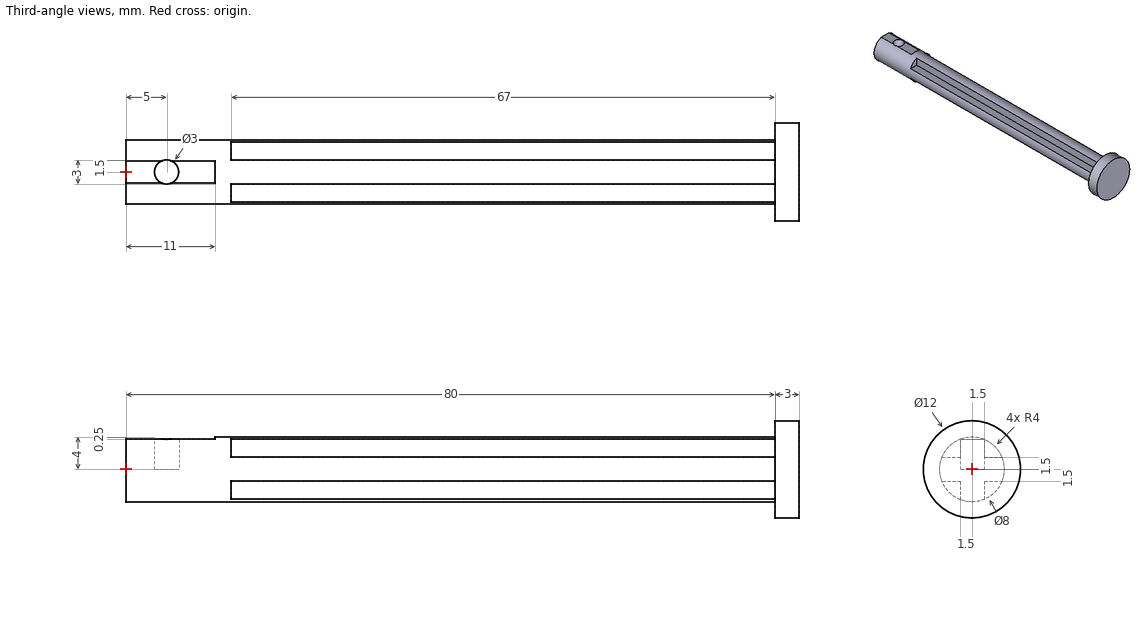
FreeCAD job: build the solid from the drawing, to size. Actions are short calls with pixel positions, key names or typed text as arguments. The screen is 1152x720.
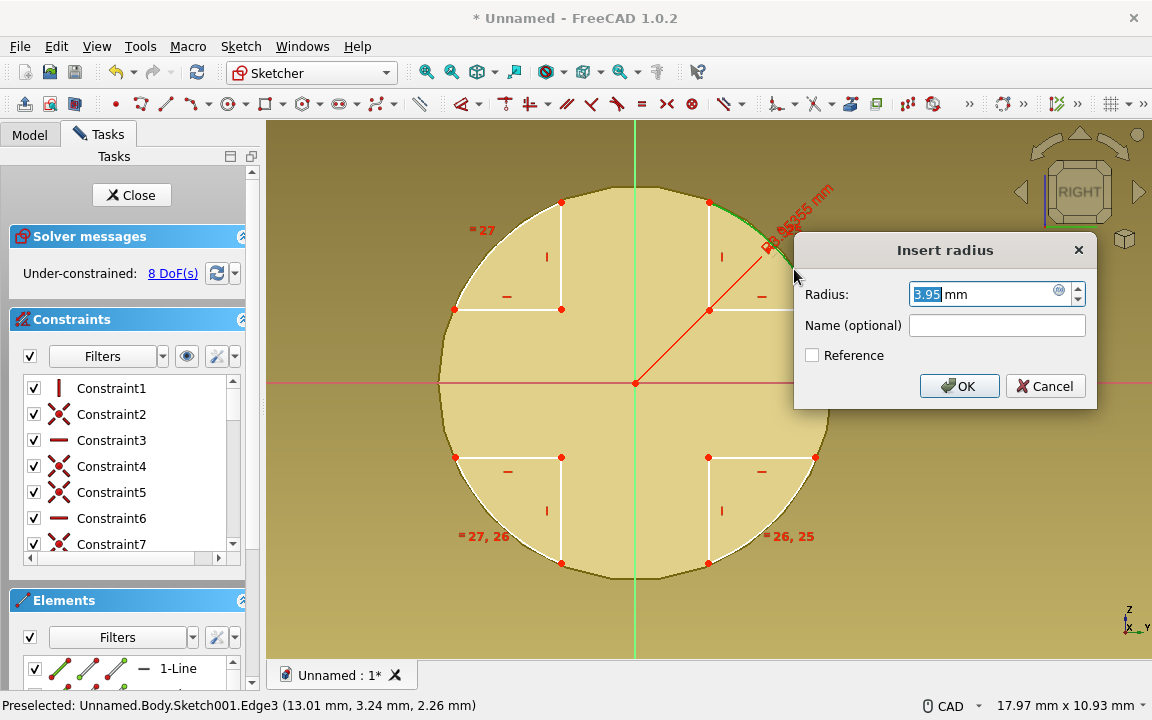
text(4)
key(Return)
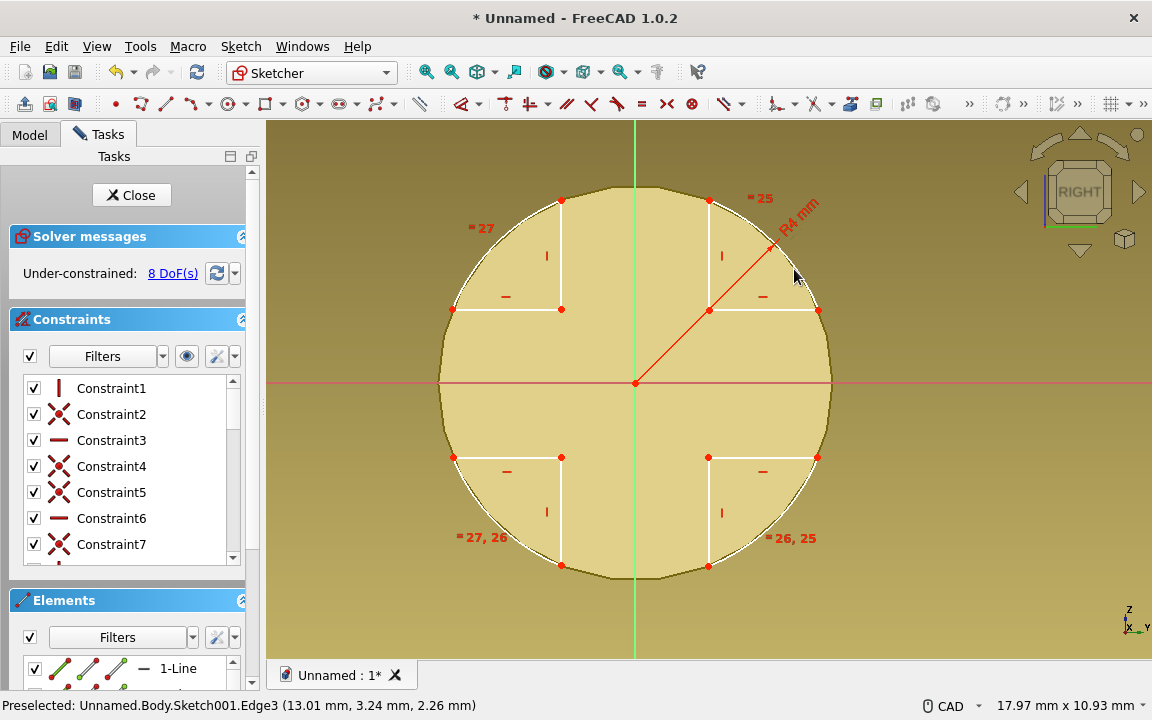
click(709, 200)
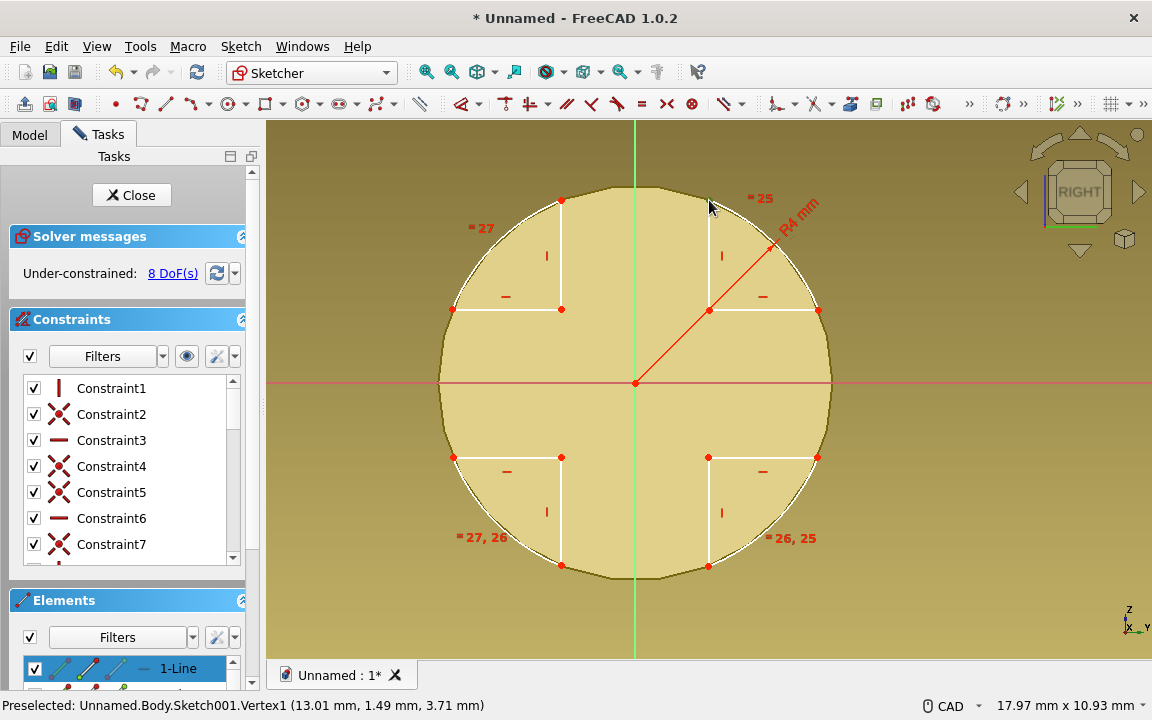
key(l)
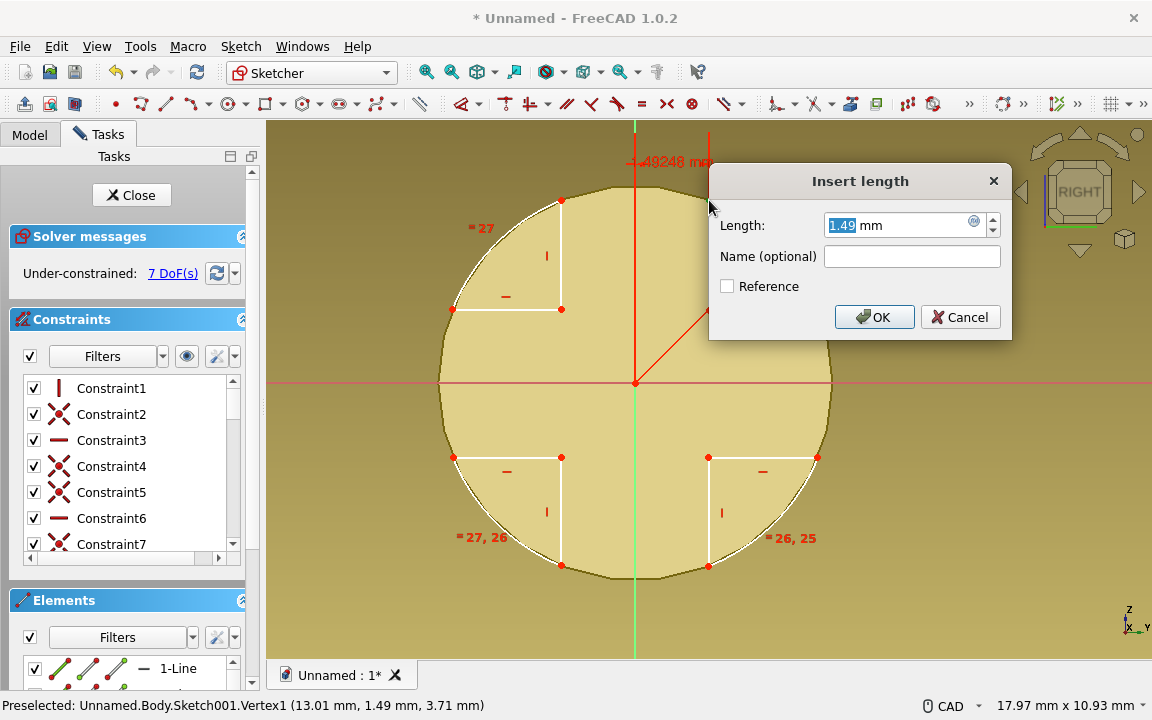
text(1.5)
key(Return)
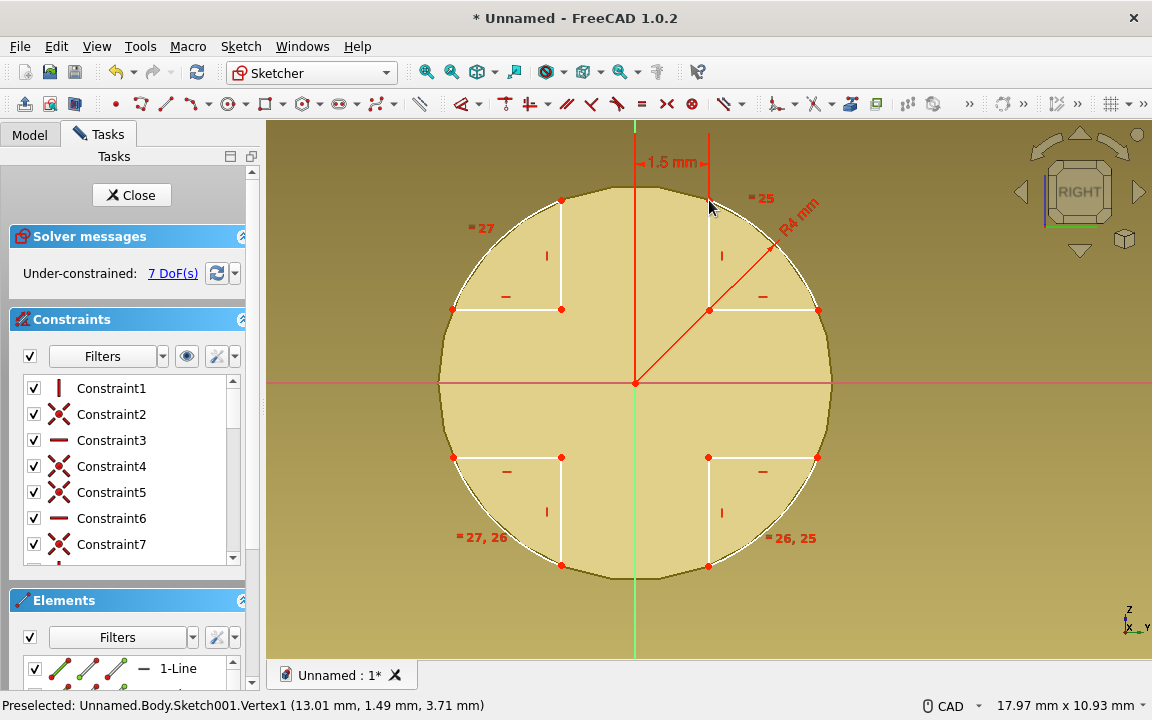
click(709, 310)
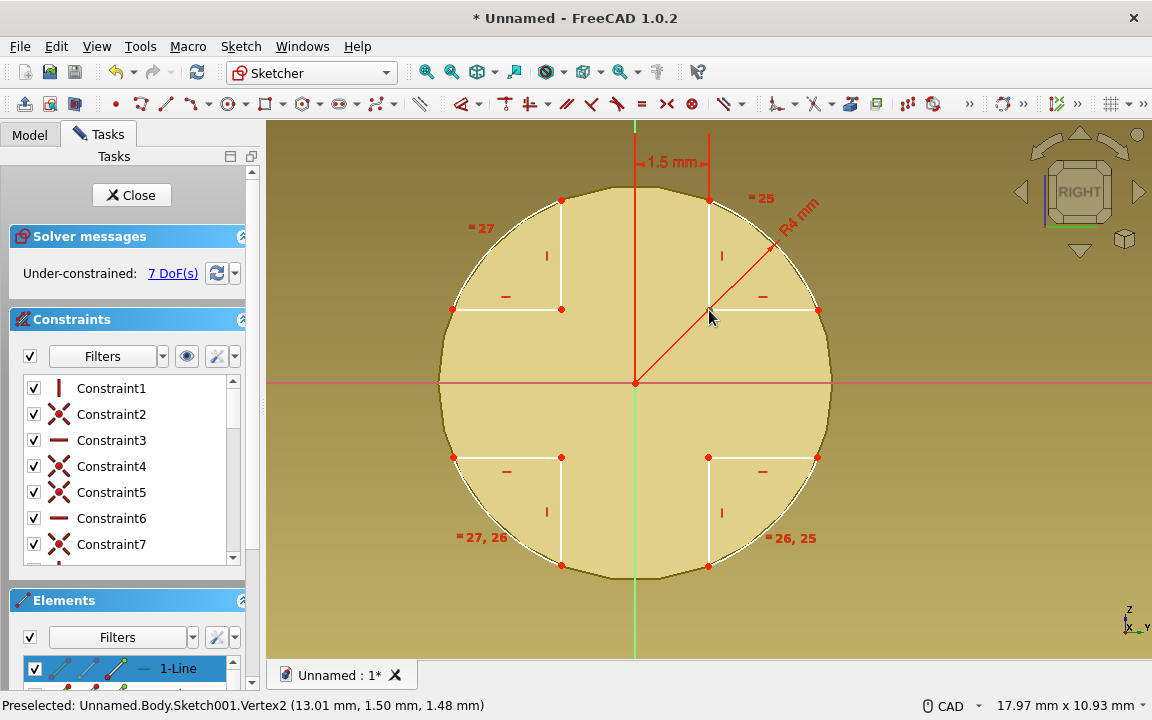
key(i)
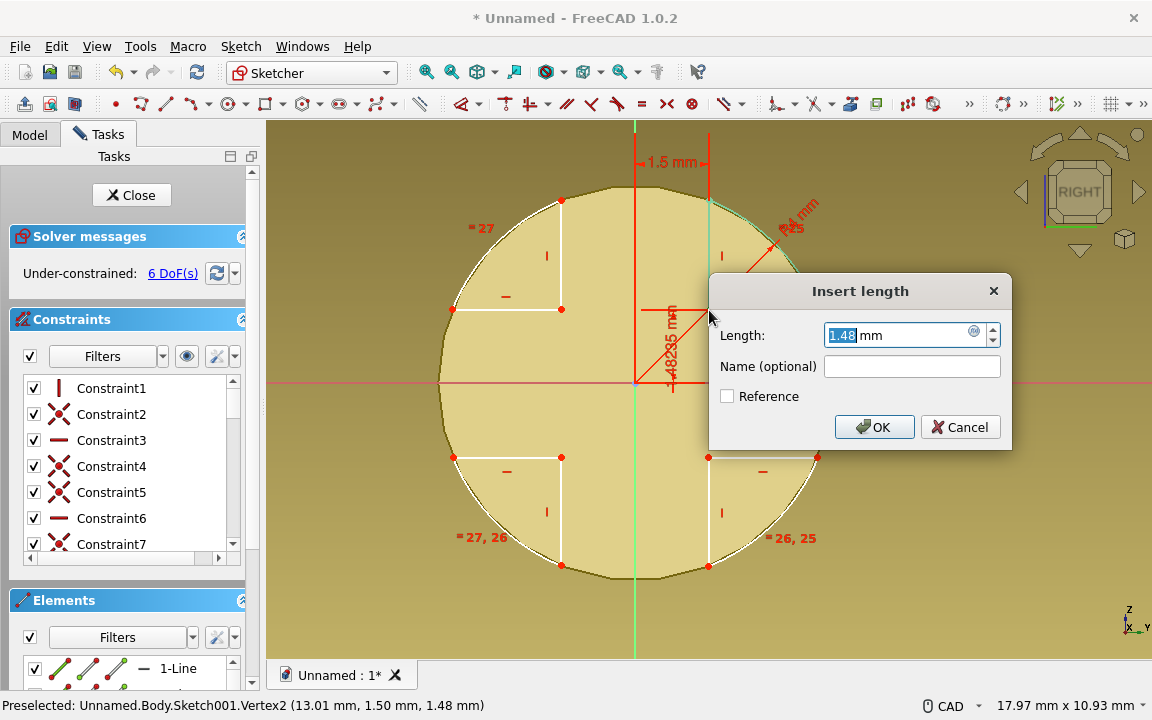
text(1.5)
key(Return)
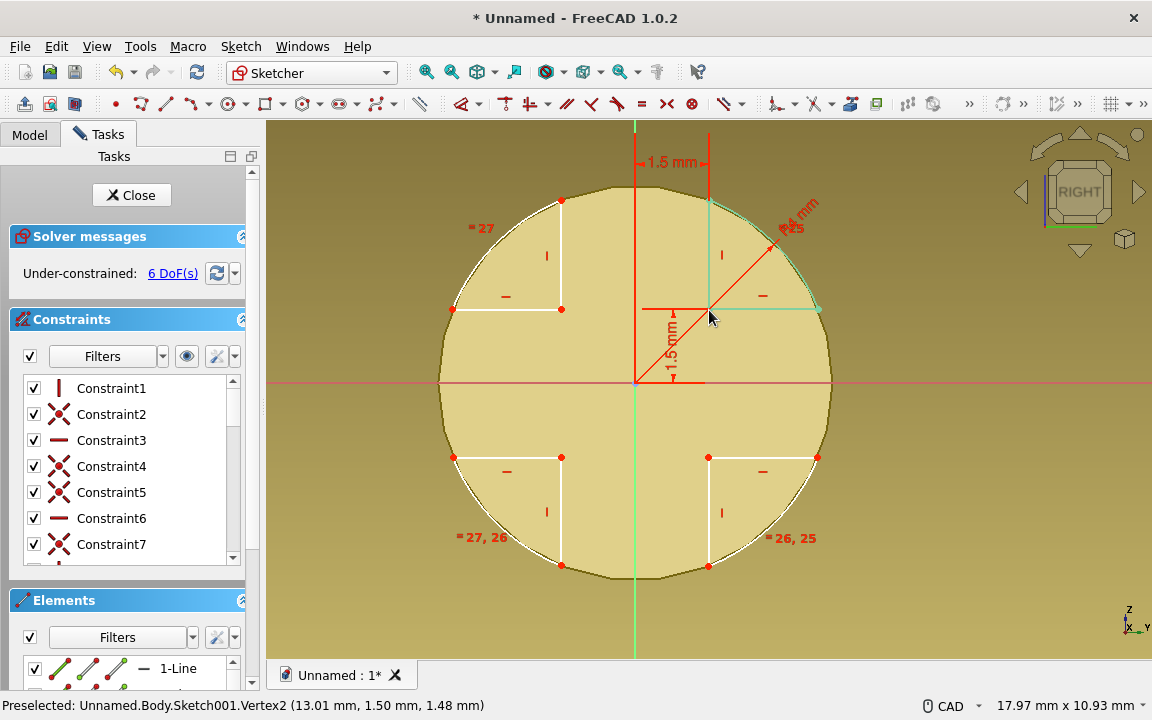
click(818, 458)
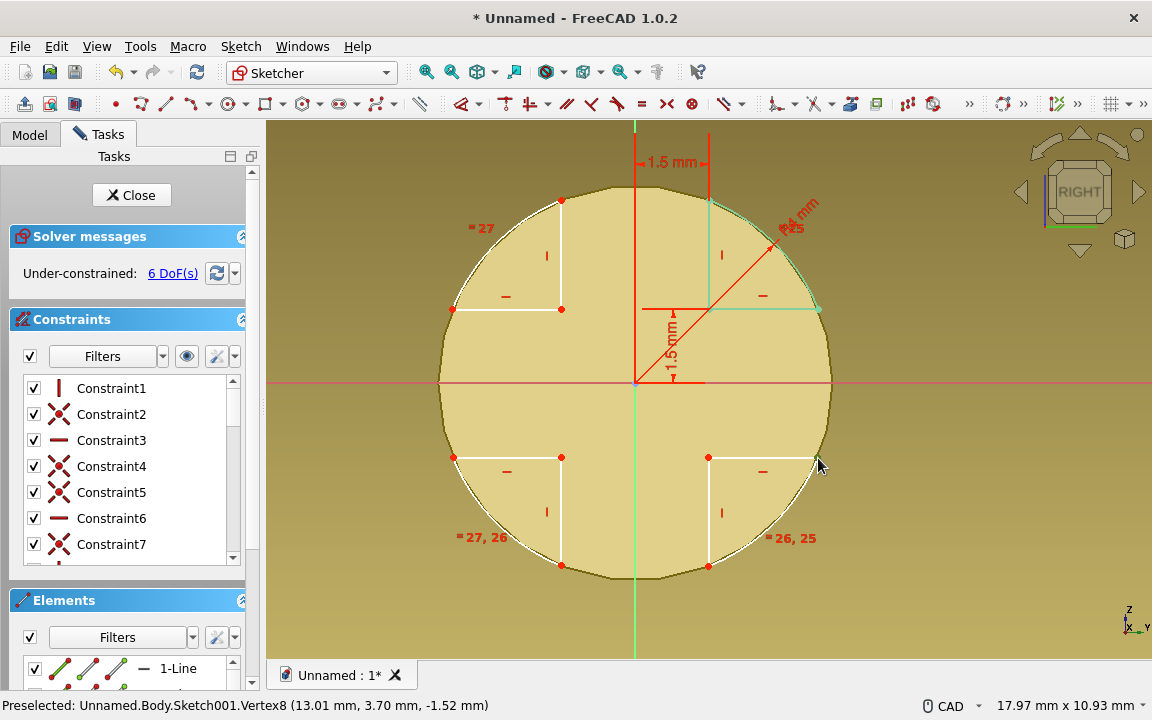
key(i)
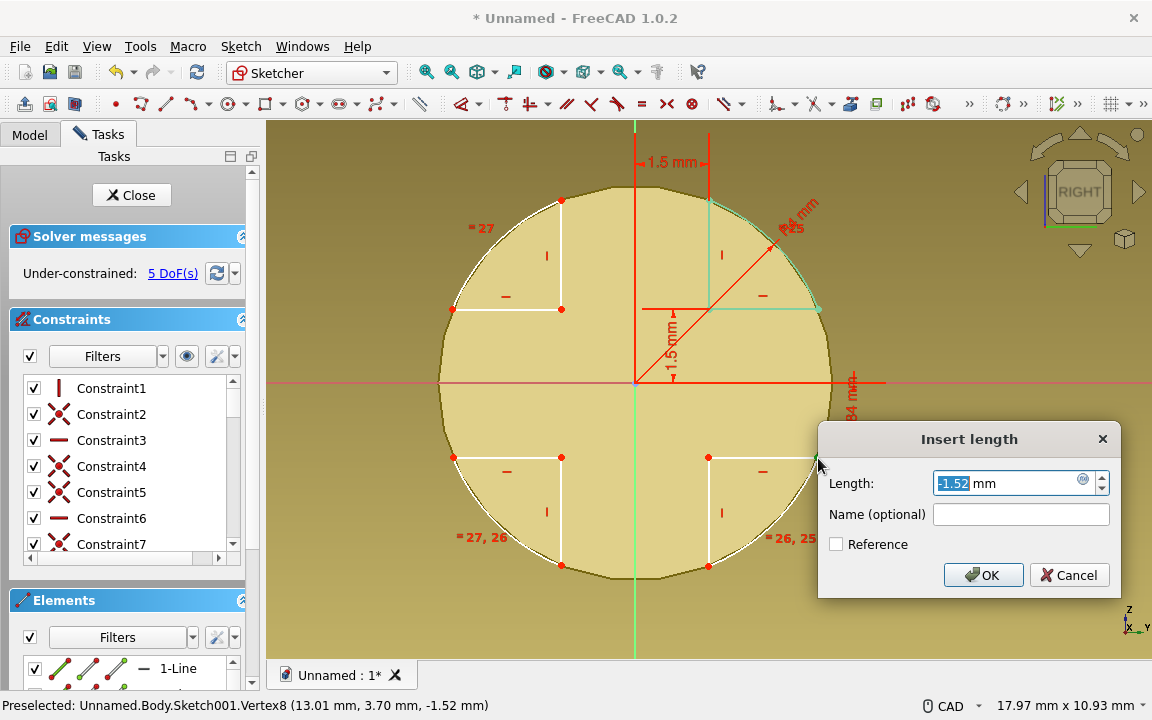
text(-1.5)
key(Return)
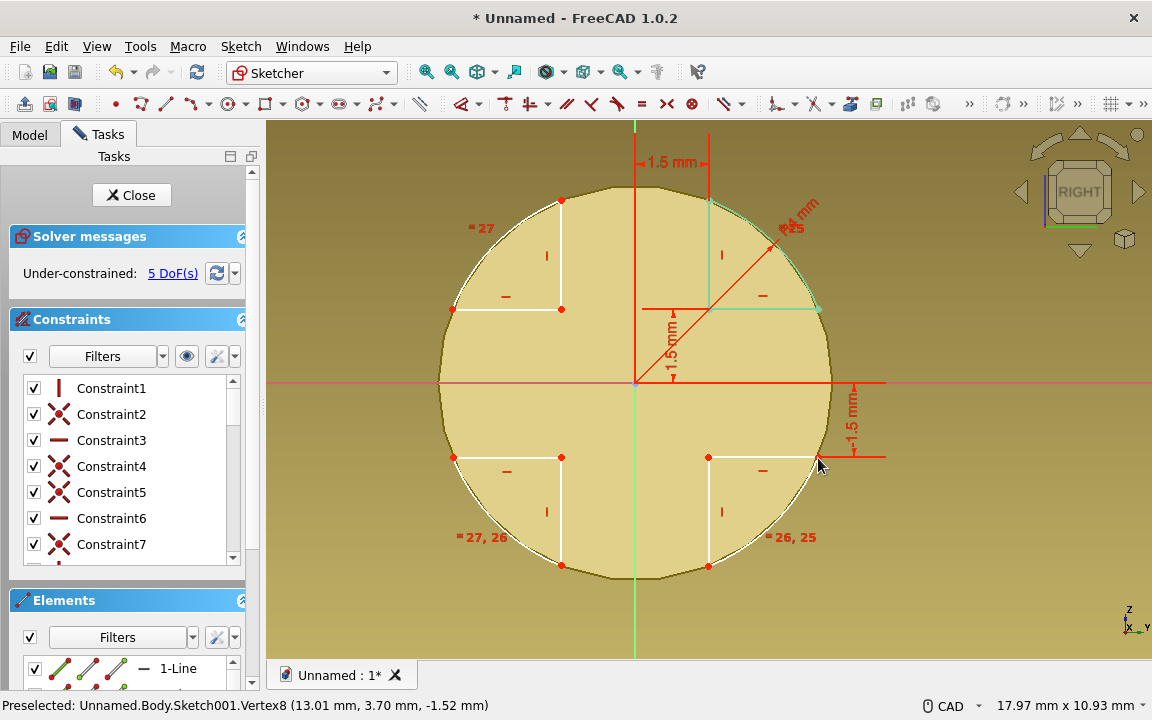
click(709, 457)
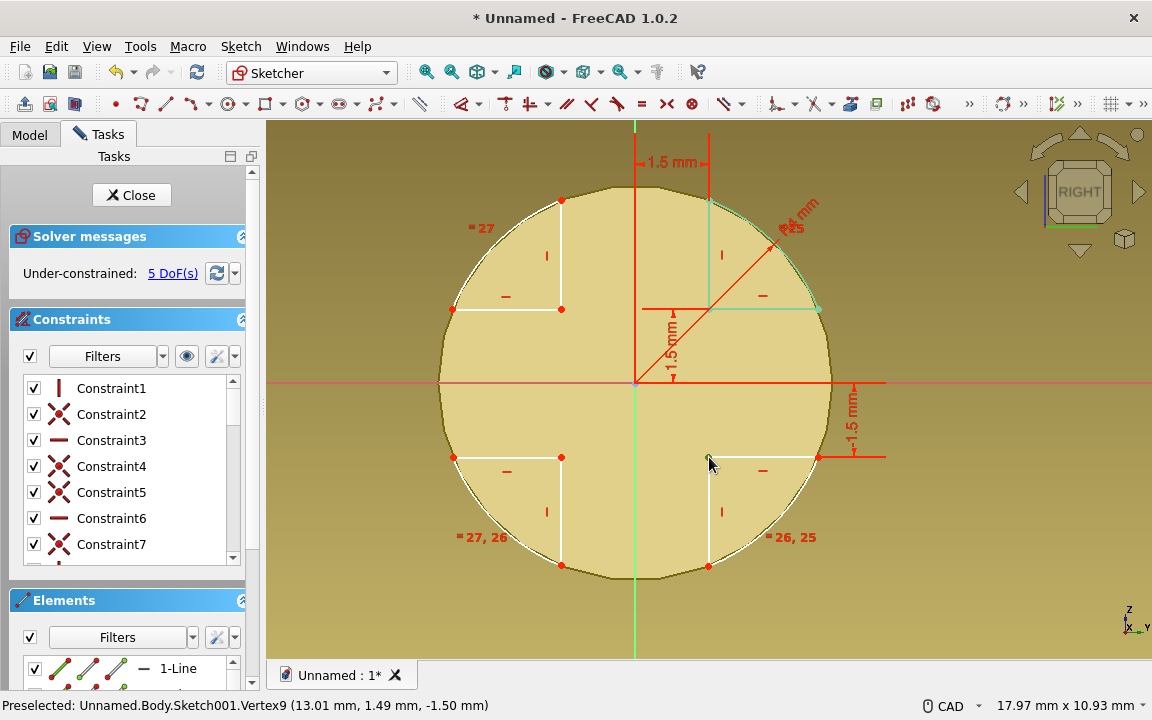
key(l)